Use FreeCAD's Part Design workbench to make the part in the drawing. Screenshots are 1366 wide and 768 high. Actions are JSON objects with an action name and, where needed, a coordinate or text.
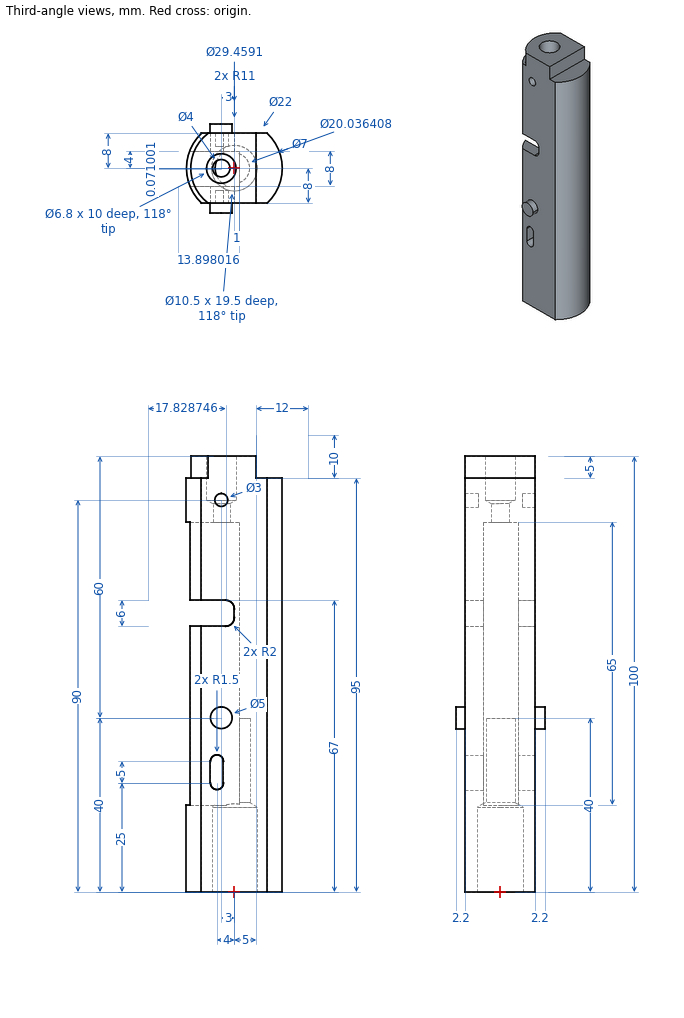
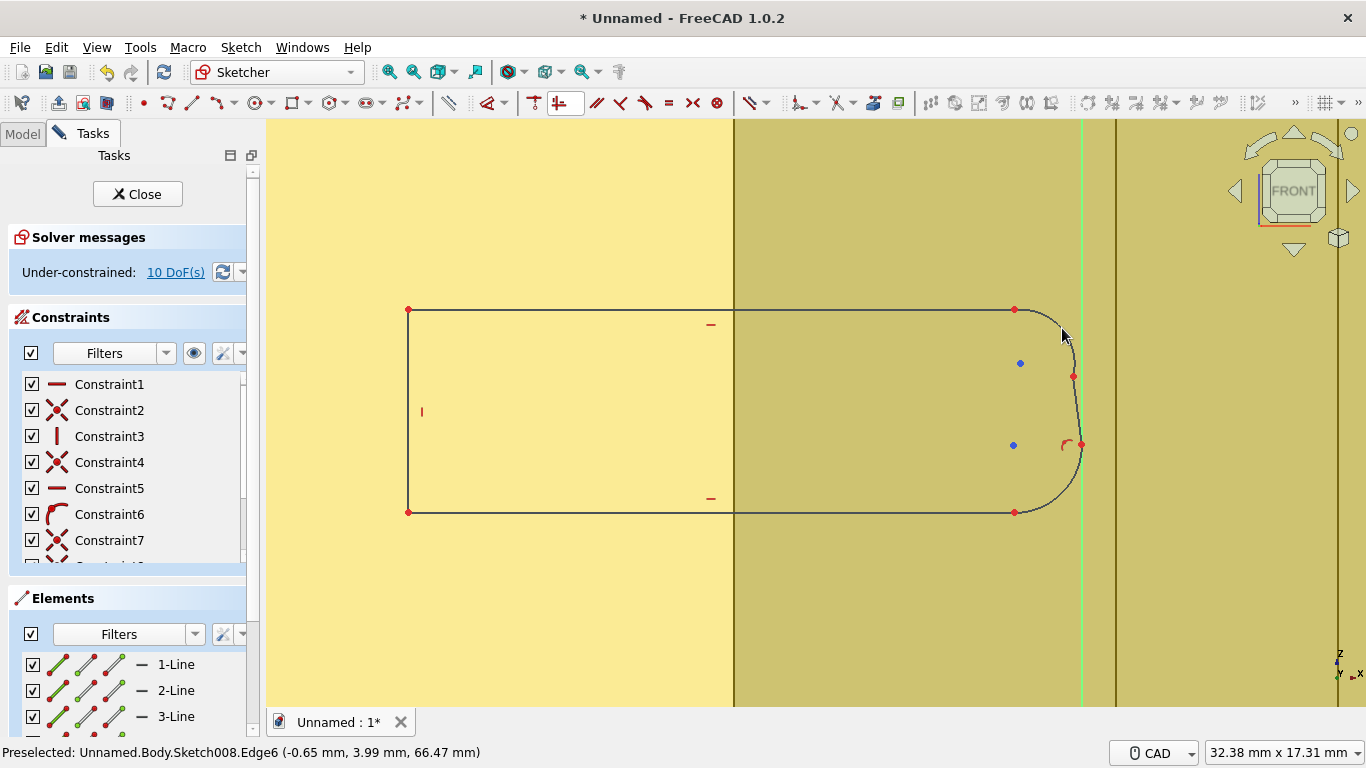
{"action": "left_click", "coordinate": [832, 310]}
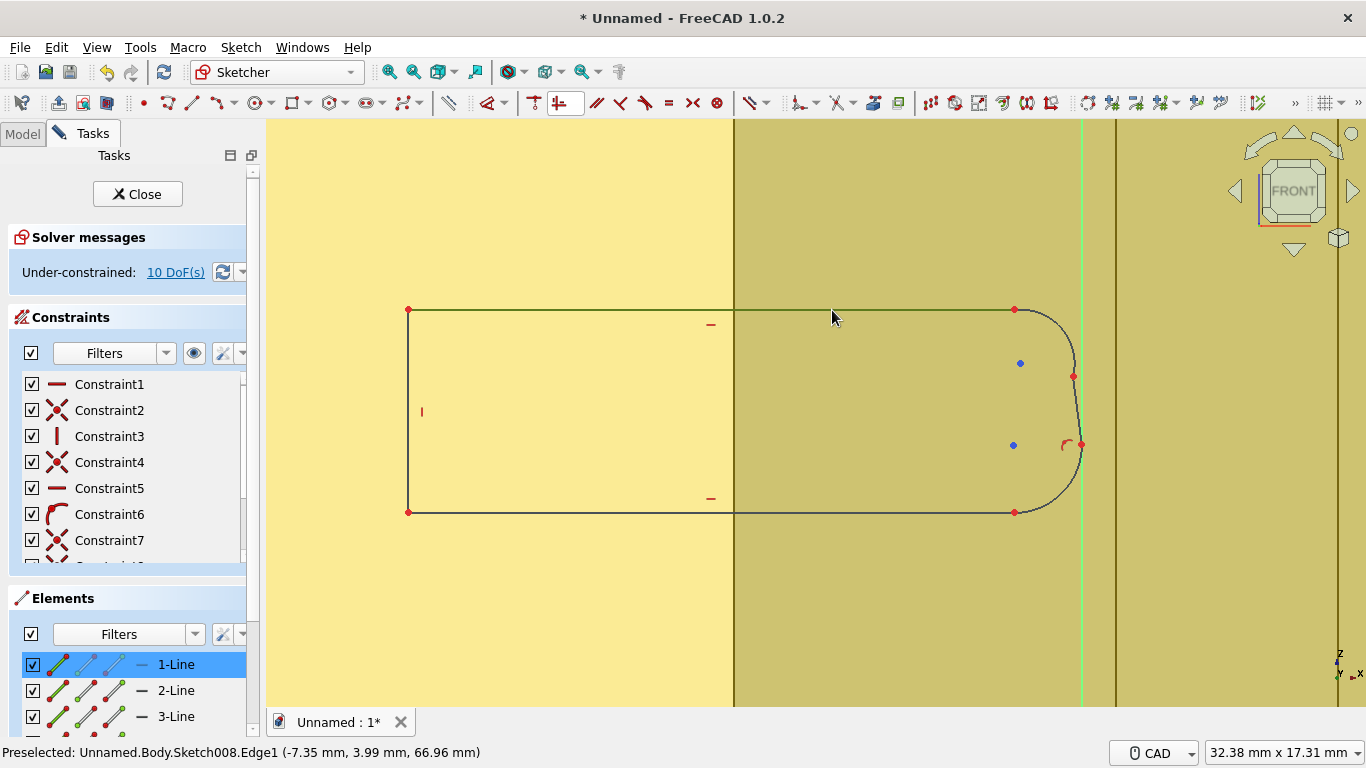
{"action": "scroll", "coordinate": [1072, 346], "scroll_direction": "up", "scroll_amount": 2}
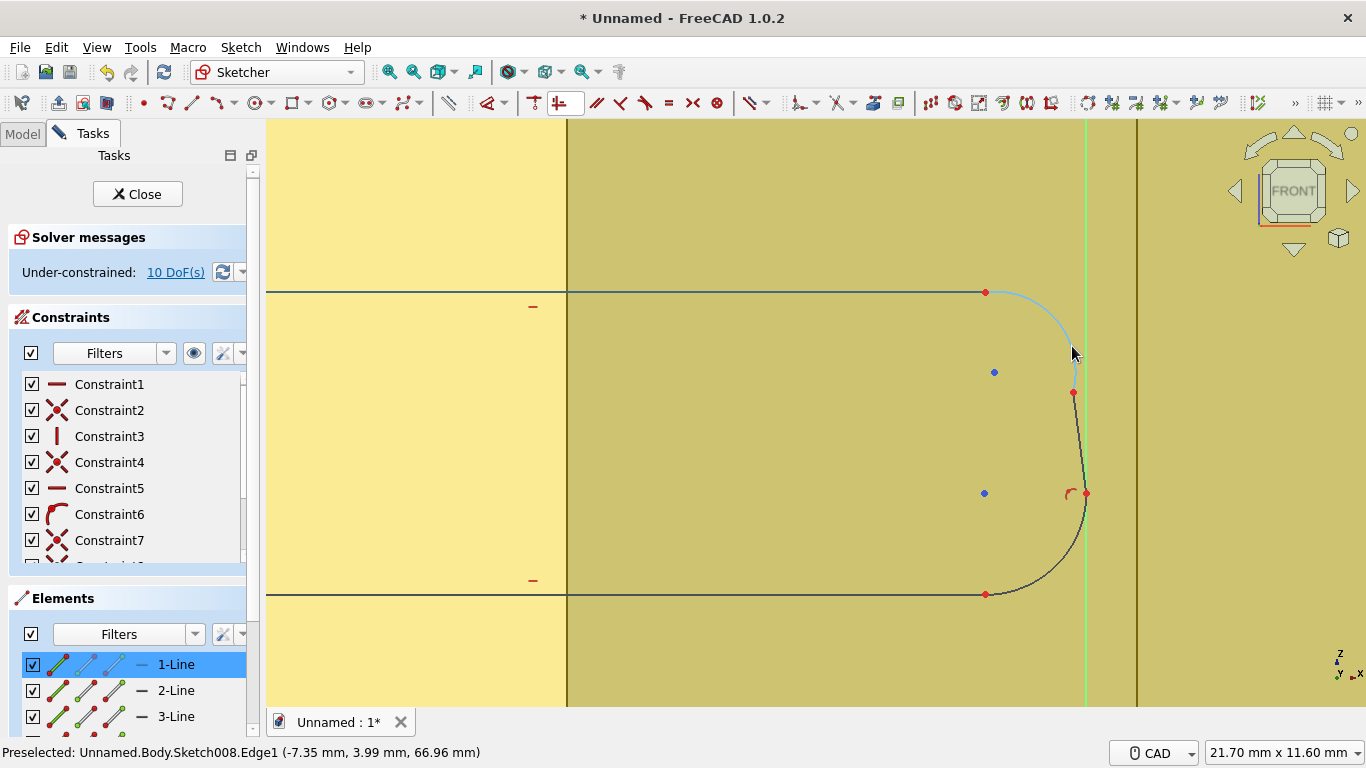
{"action": "left_click", "coordinate": [1071, 346]}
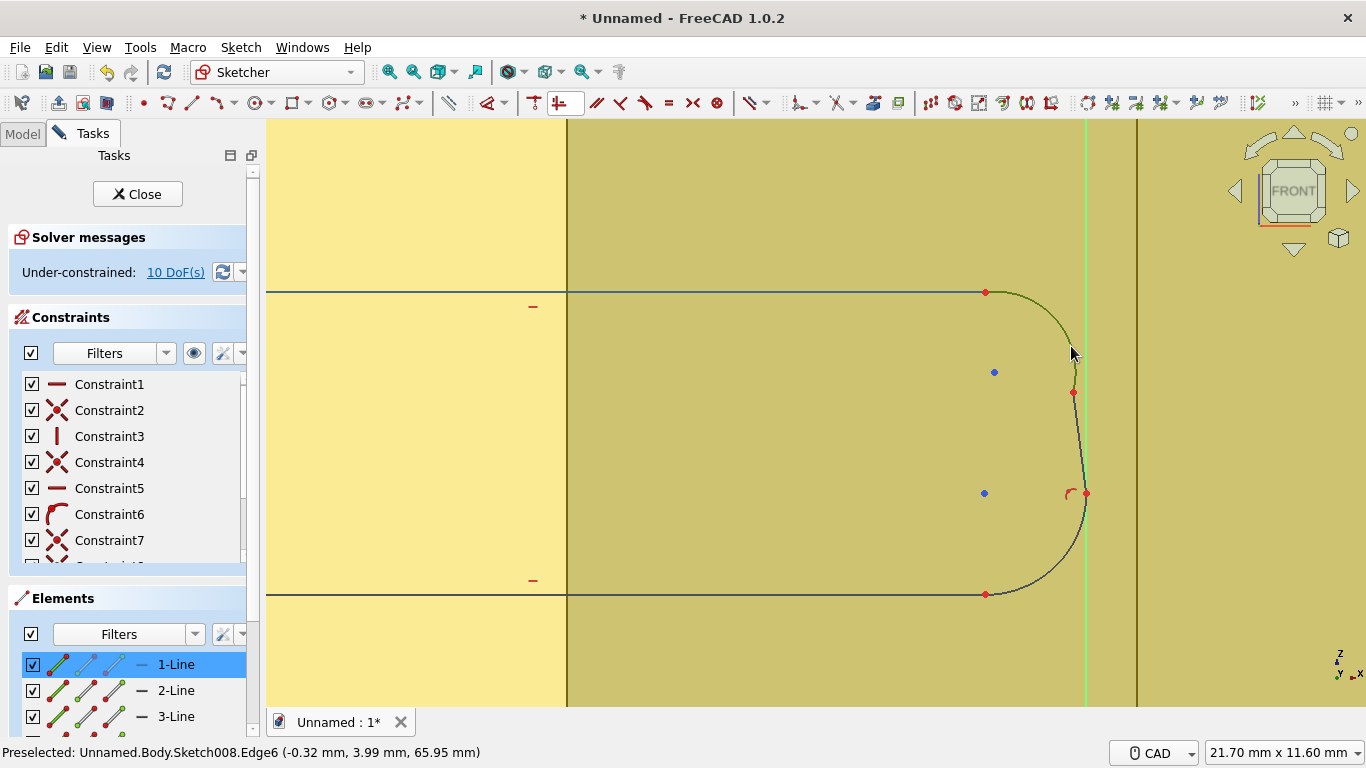
{"action": "key", "text": "t"}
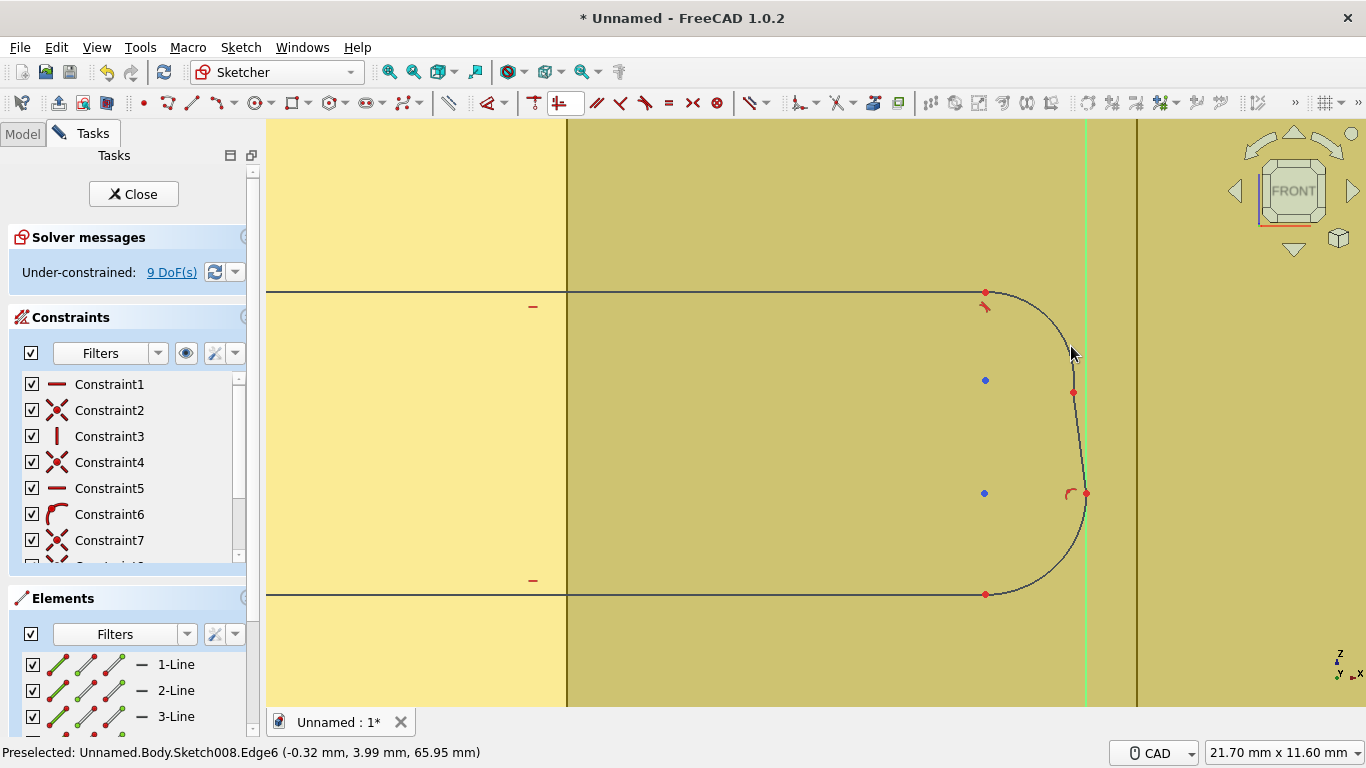
{"action": "left_click", "coordinate": [352, 595]}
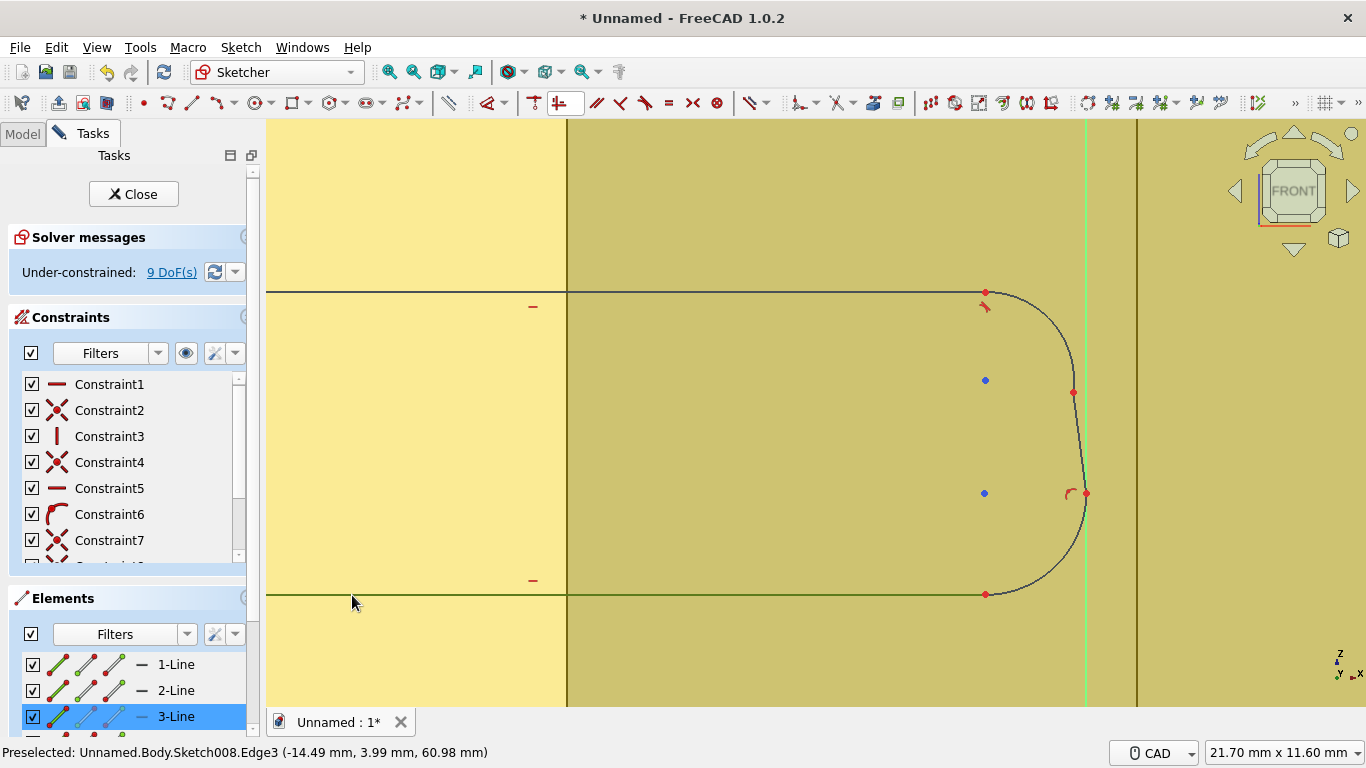
{"action": "left_click", "coordinate": [1031, 584]}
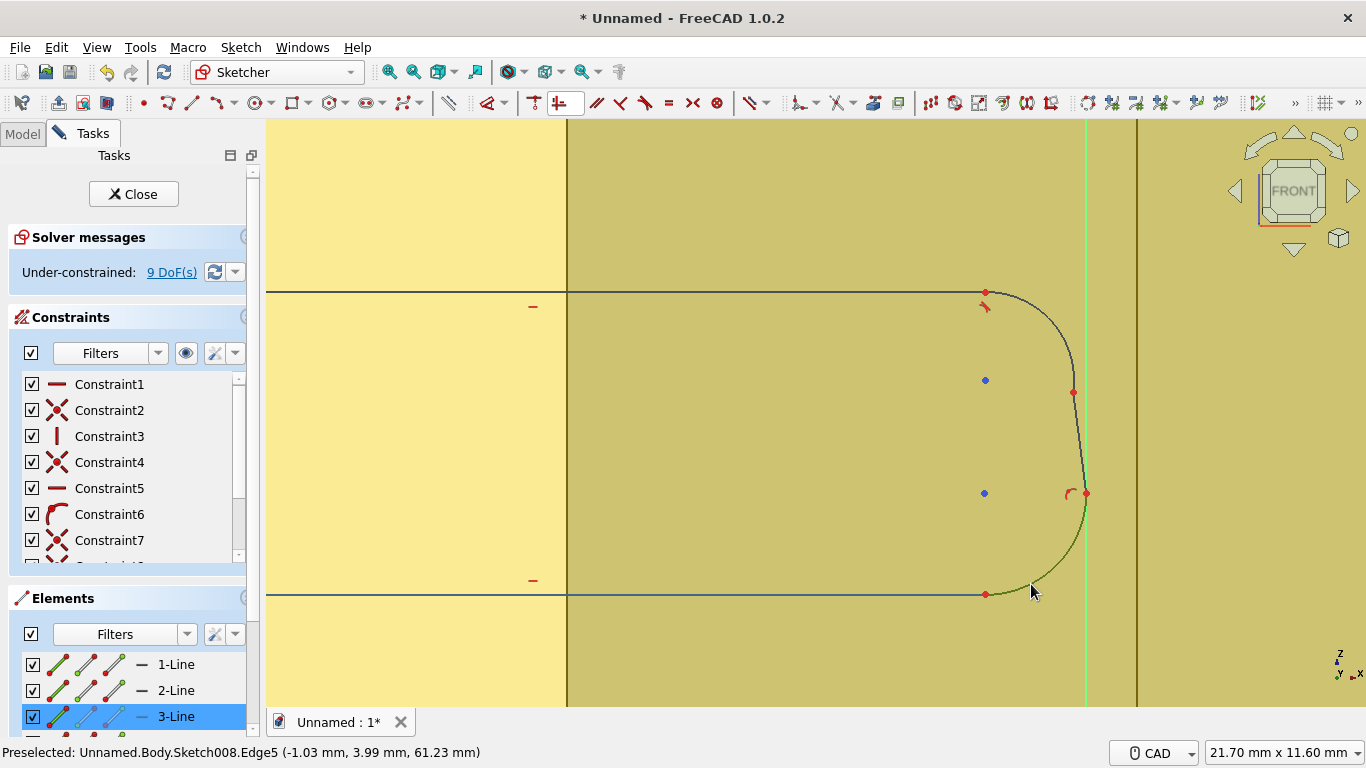
{"action": "key", "text": "t"}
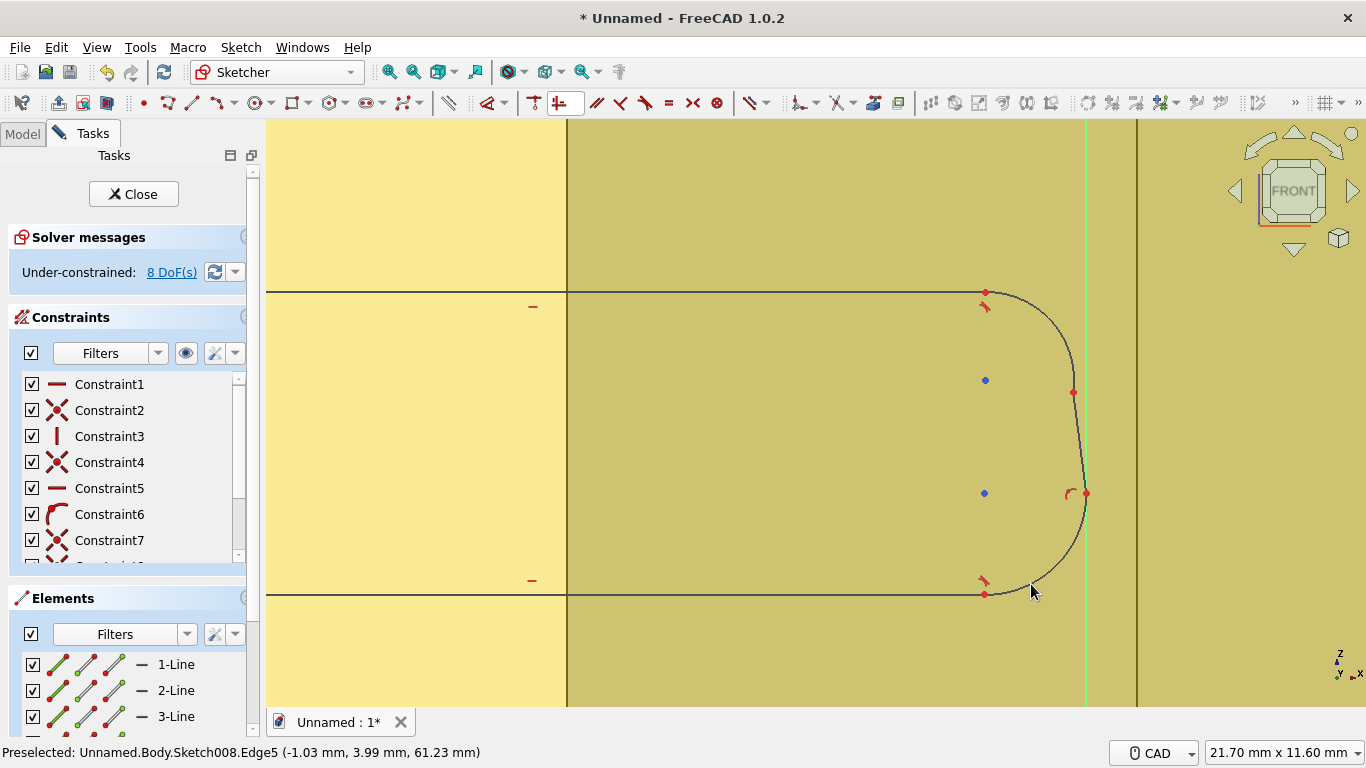
{"action": "left_click", "coordinate": [1082, 463]}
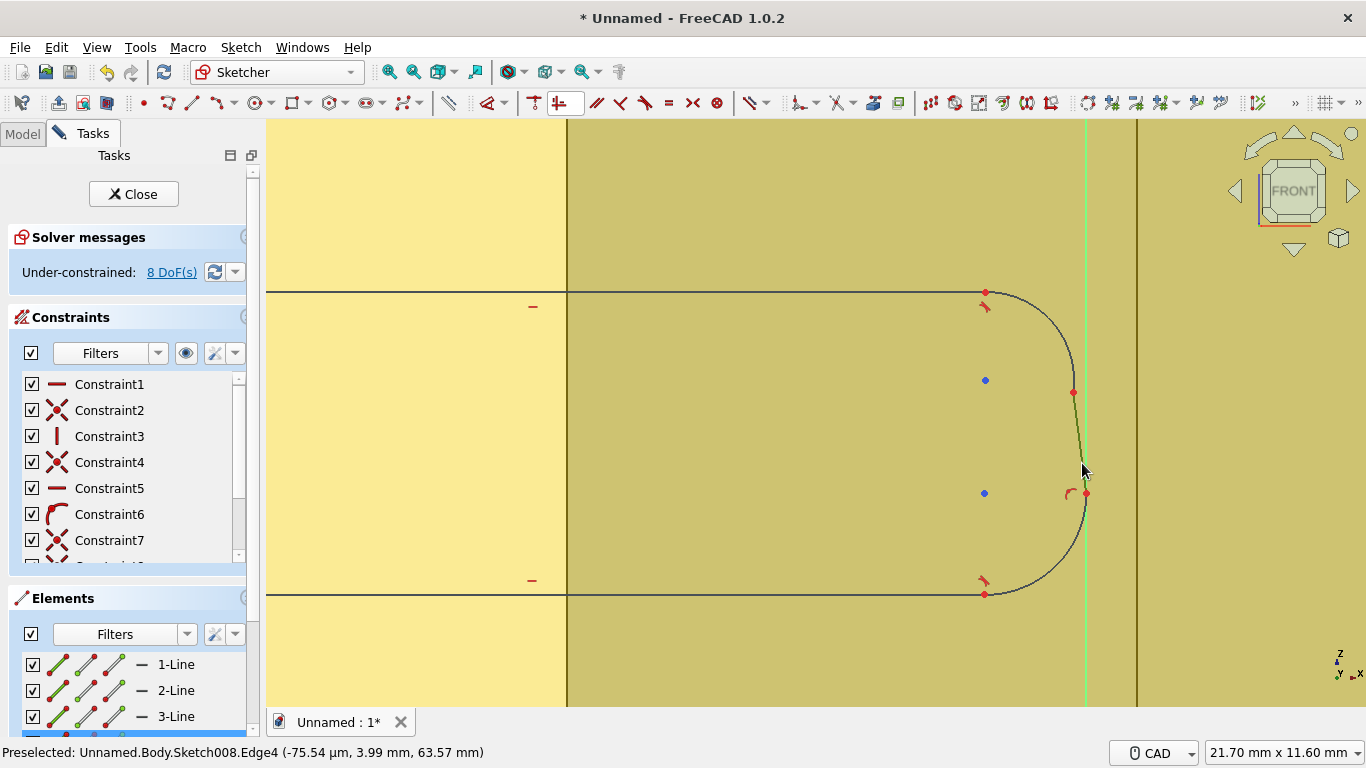
{"action": "left_click", "coordinate": [1031, 584]}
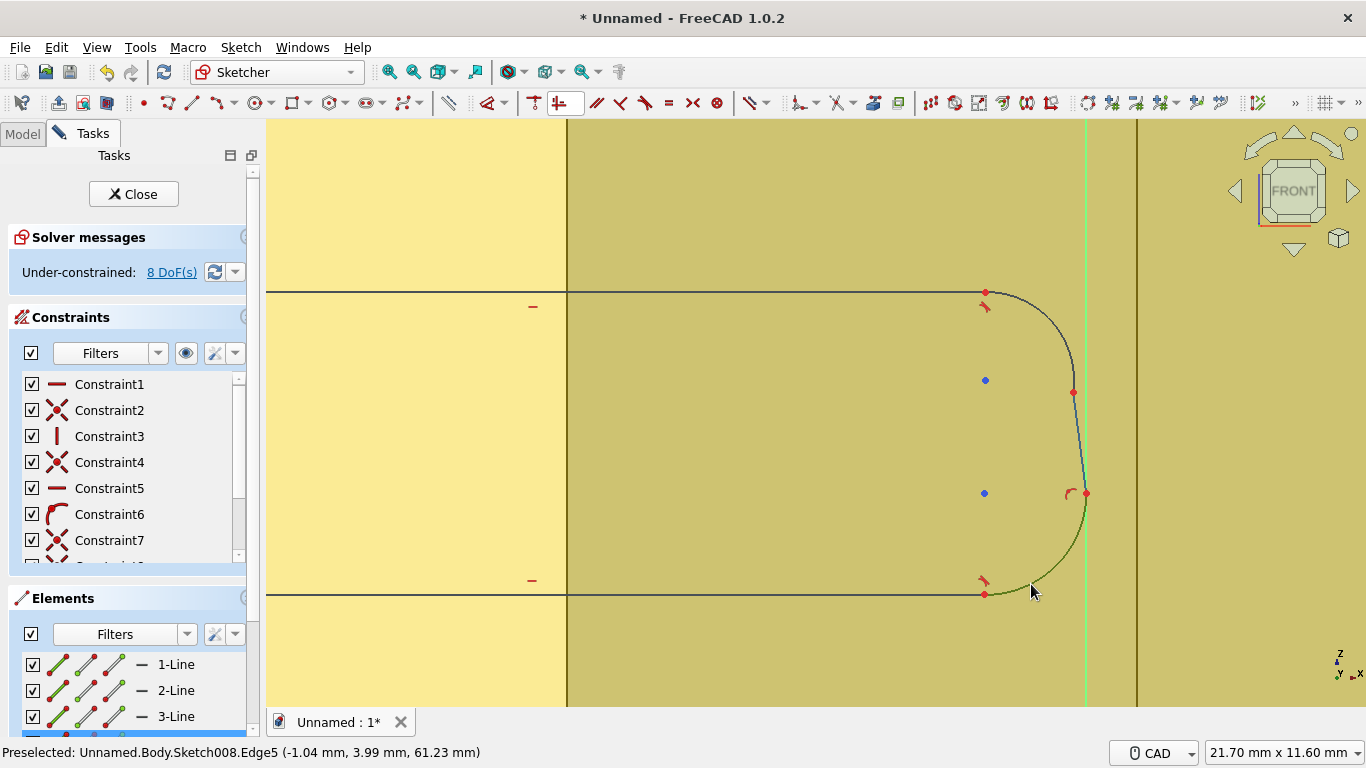
{"action": "key", "text": "t"}